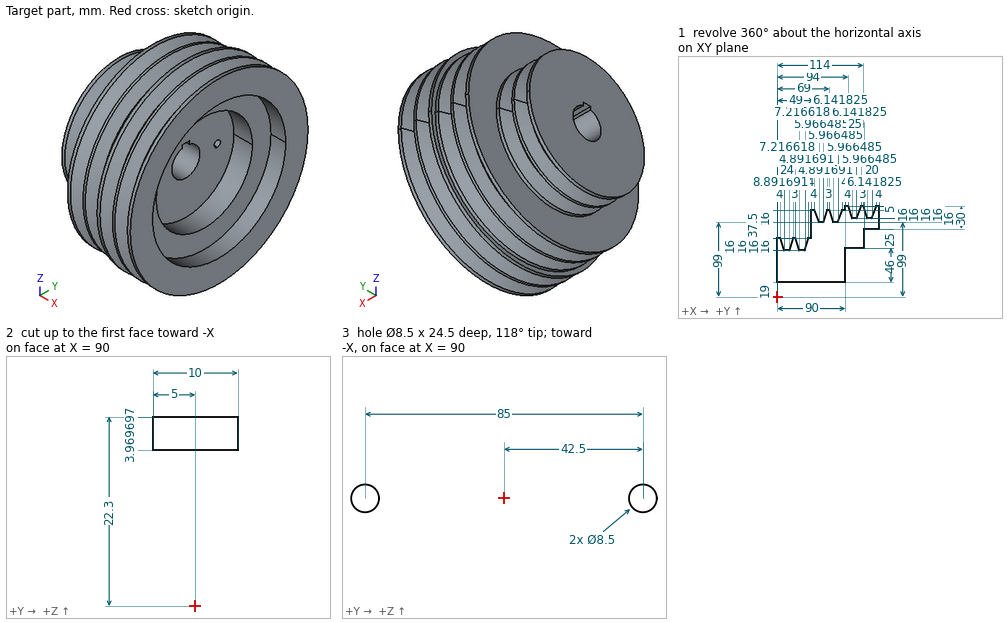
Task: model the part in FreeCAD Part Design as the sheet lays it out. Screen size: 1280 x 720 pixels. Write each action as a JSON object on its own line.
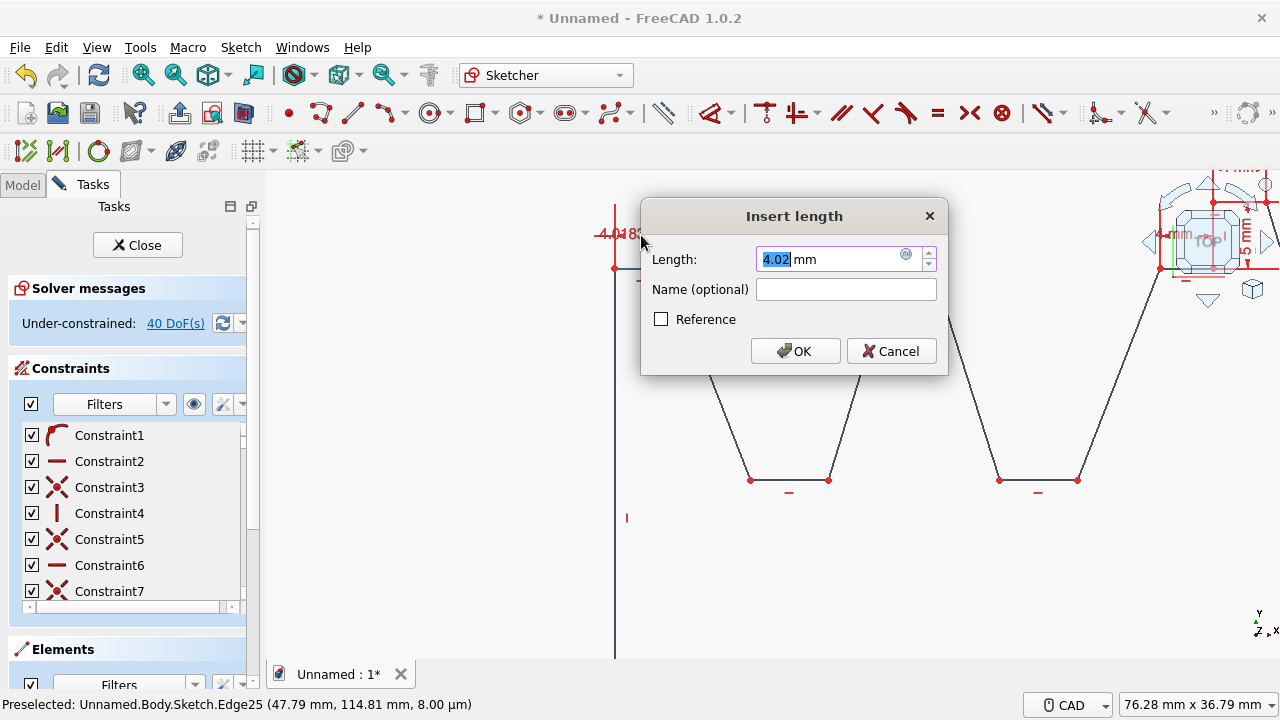
{"action": "type", "text": "4"}
{"action": "key", "text": "Return"}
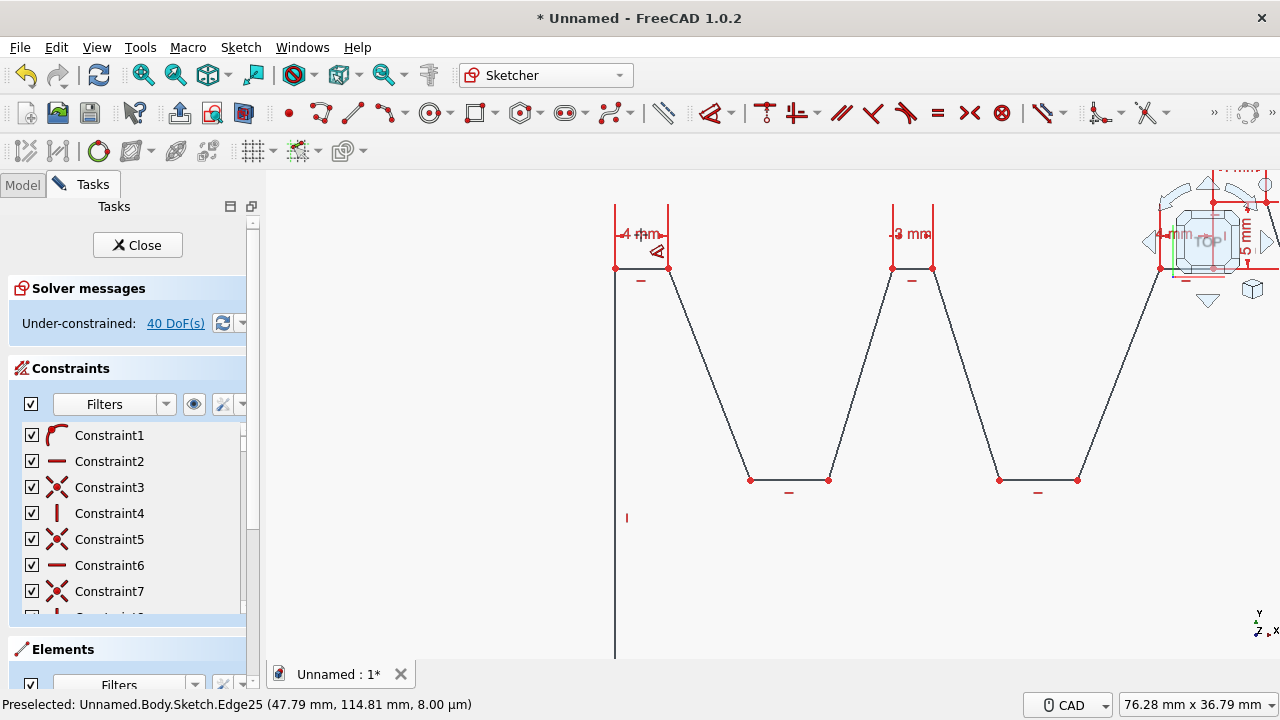
{"action": "scroll", "coordinate": [652, 267], "scroll_direction": "down", "scroll_amount": 8}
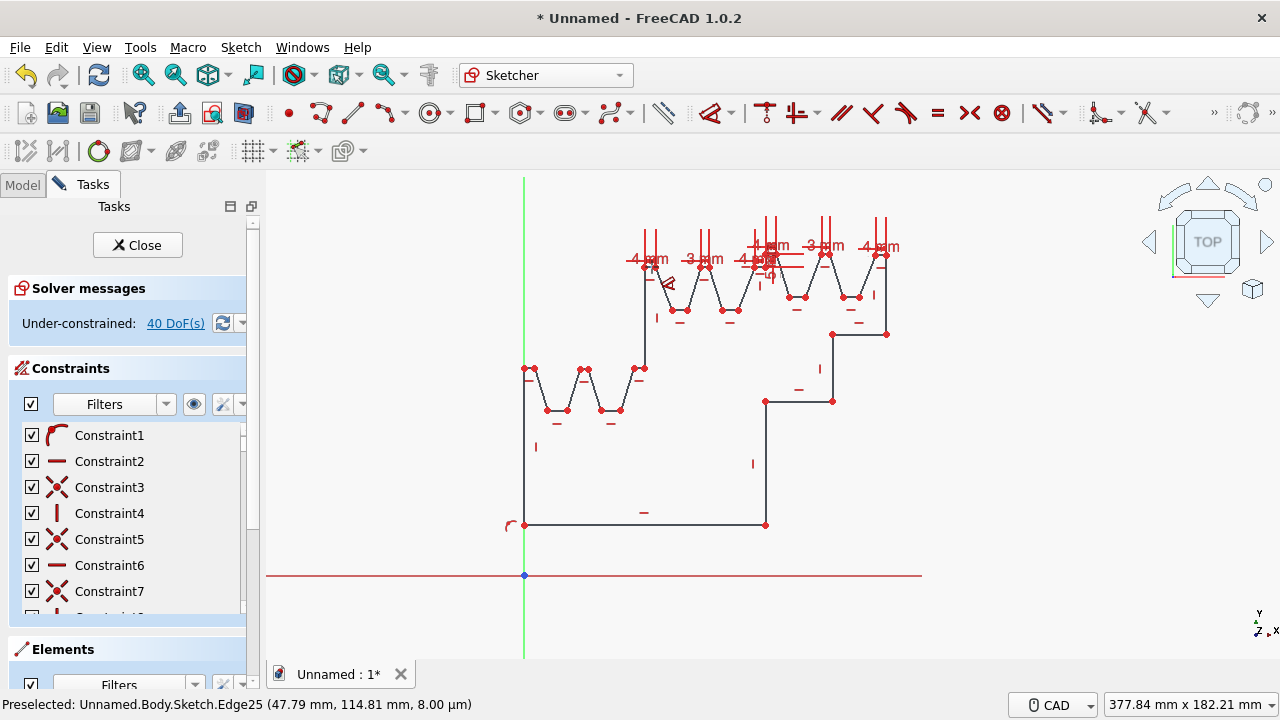
{"action": "scroll", "coordinate": [642, 368], "scroll_direction": "up", "scroll_amount": 8}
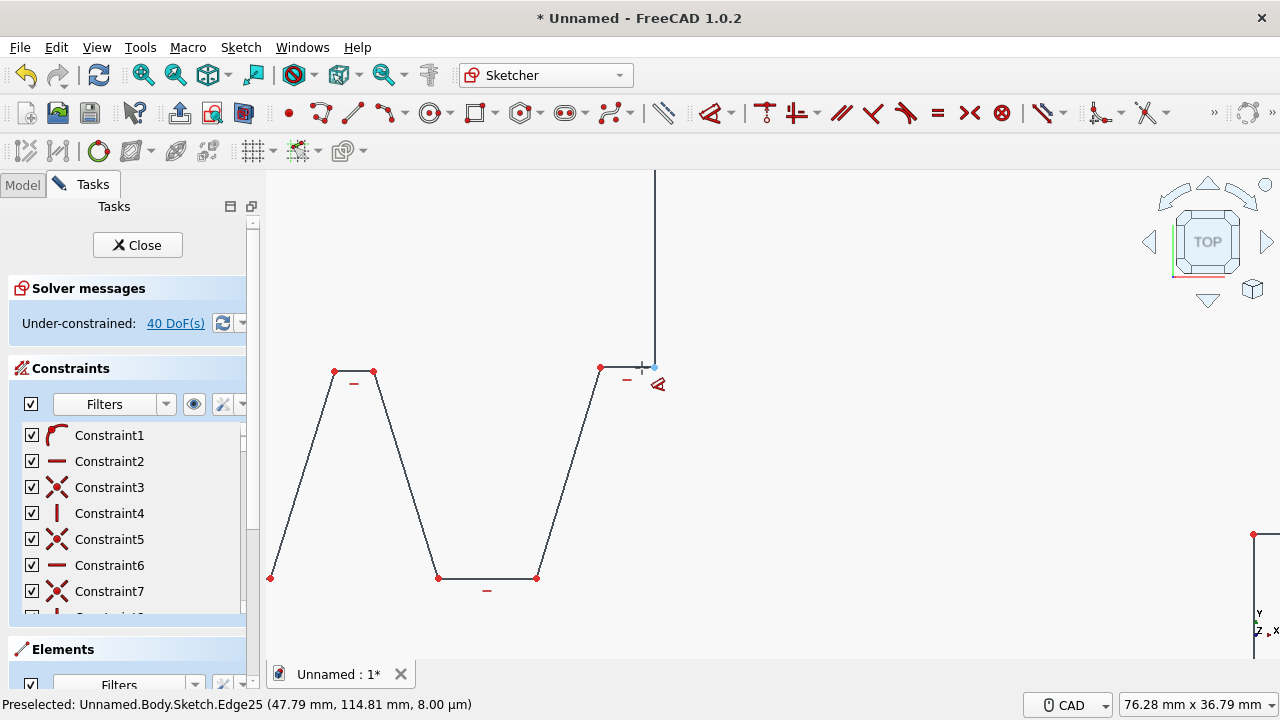
{"action": "left_click", "coordinate": [638, 367]}
{"action": "left_click", "coordinate": [628, 333]}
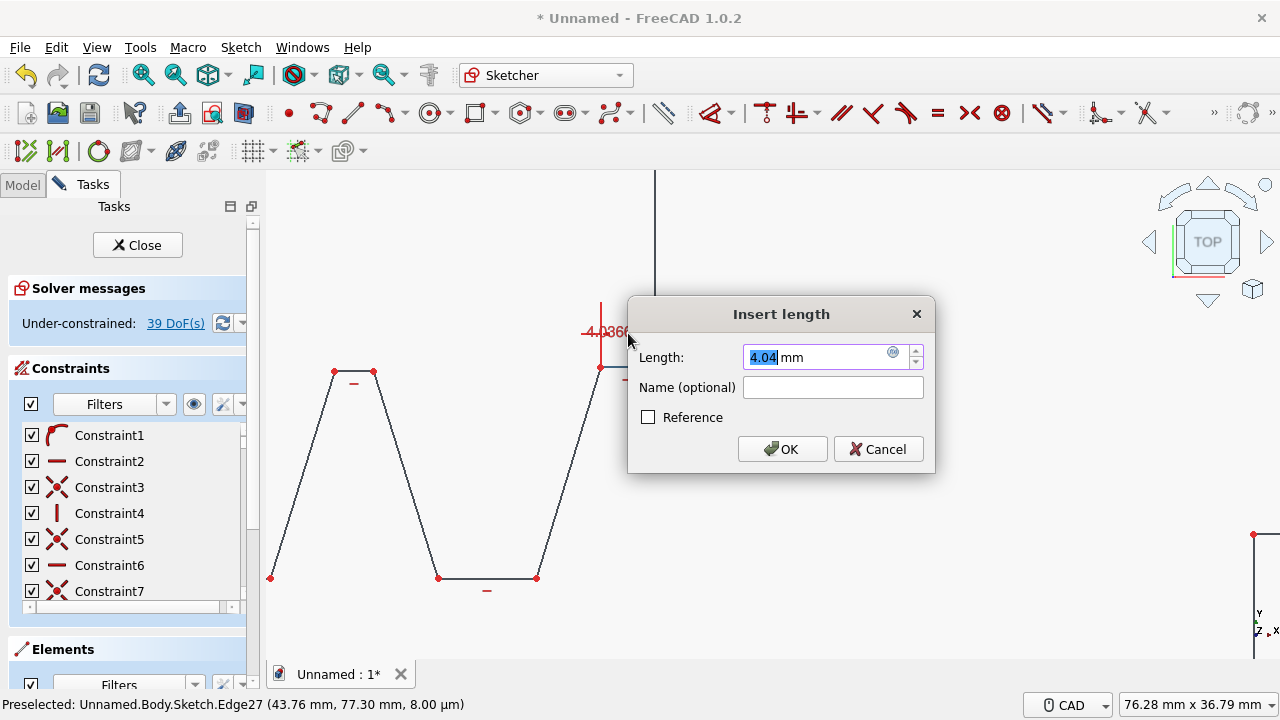
{"action": "type", "text": "4"}
{"action": "key", "text": "Return"}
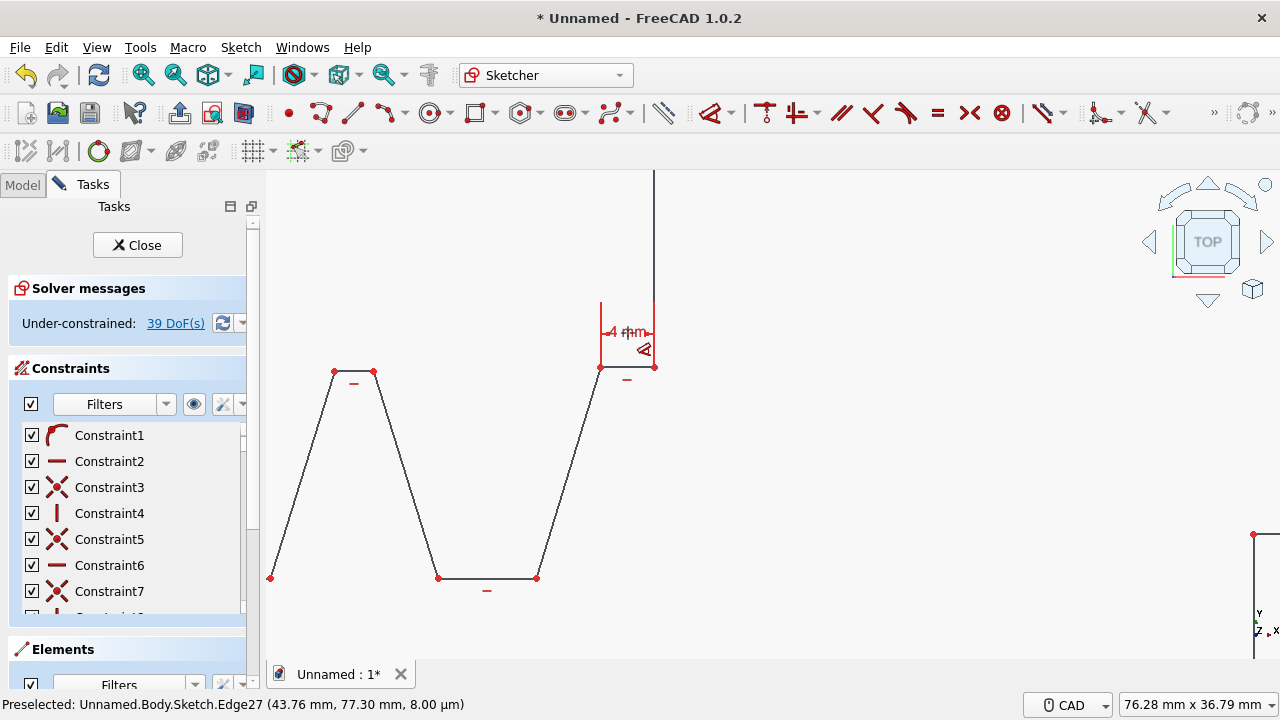
{"action": "left_click", "coordinate": [362, 371]}
{"action": "left_click", "coordinate": [354, 337]}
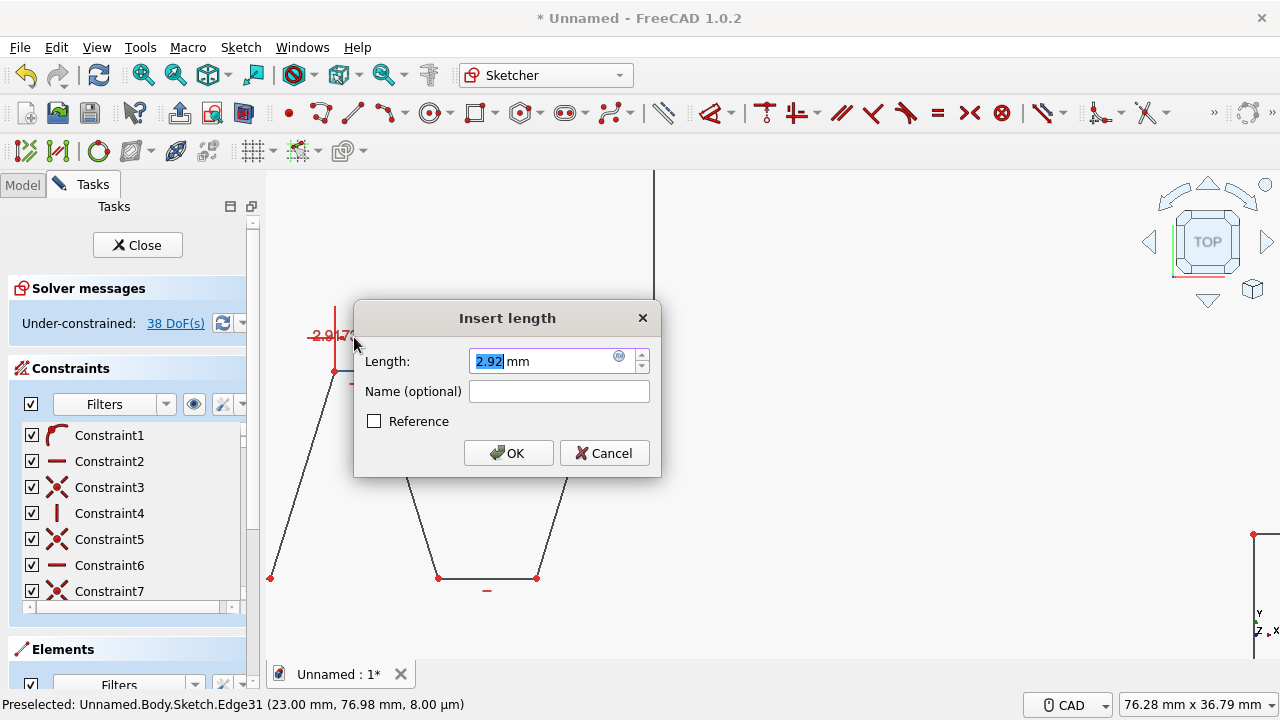
{"action": "type", "text": "3"}
{"action": "key", "text": "Return"}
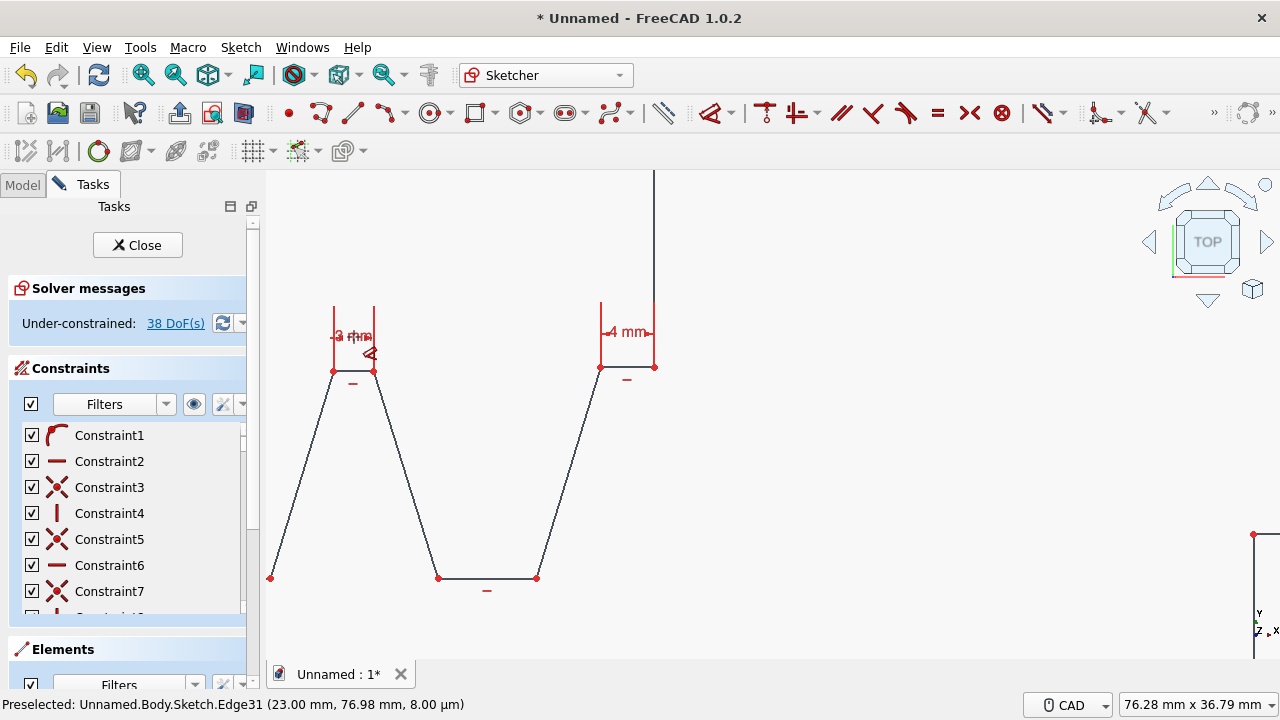
{"action": "scroll", "coordinate": [641, 368], "scroll_direction": "down", "scroll_amount": 8}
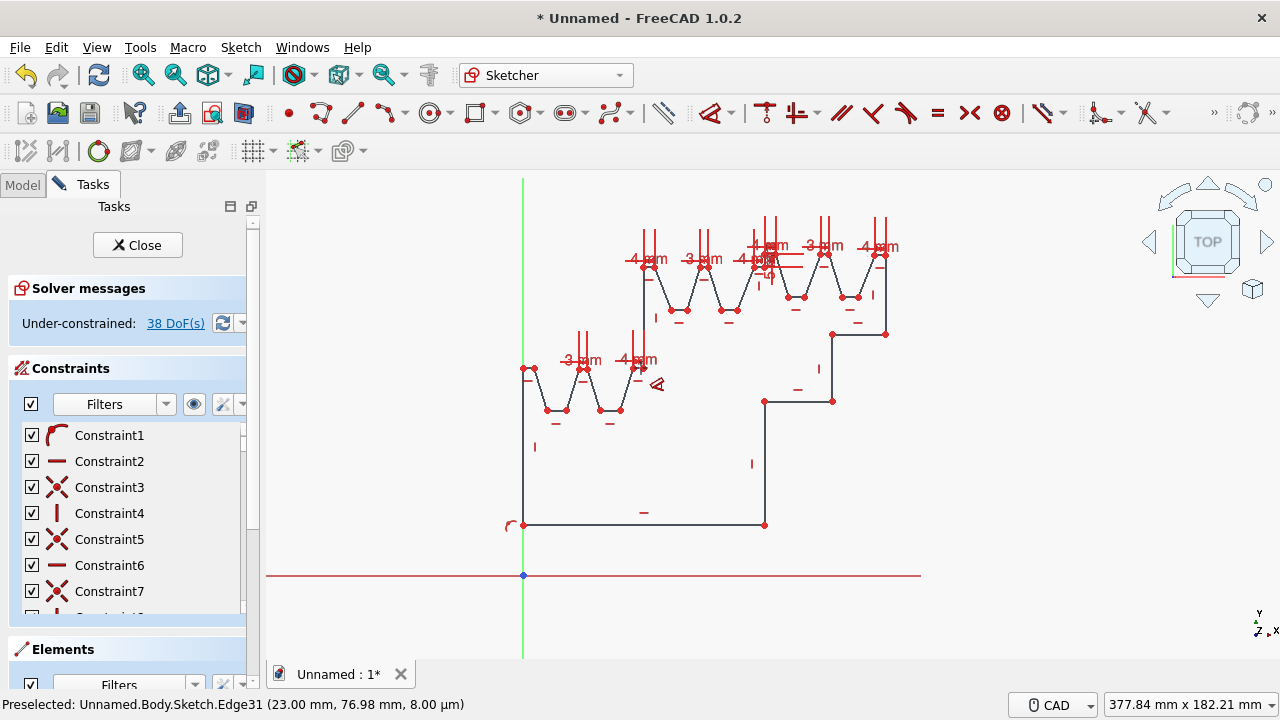
{"action": "scroll", "coordinate": [531, 368], "scroll_direction": "up", "scroll_amount": 8}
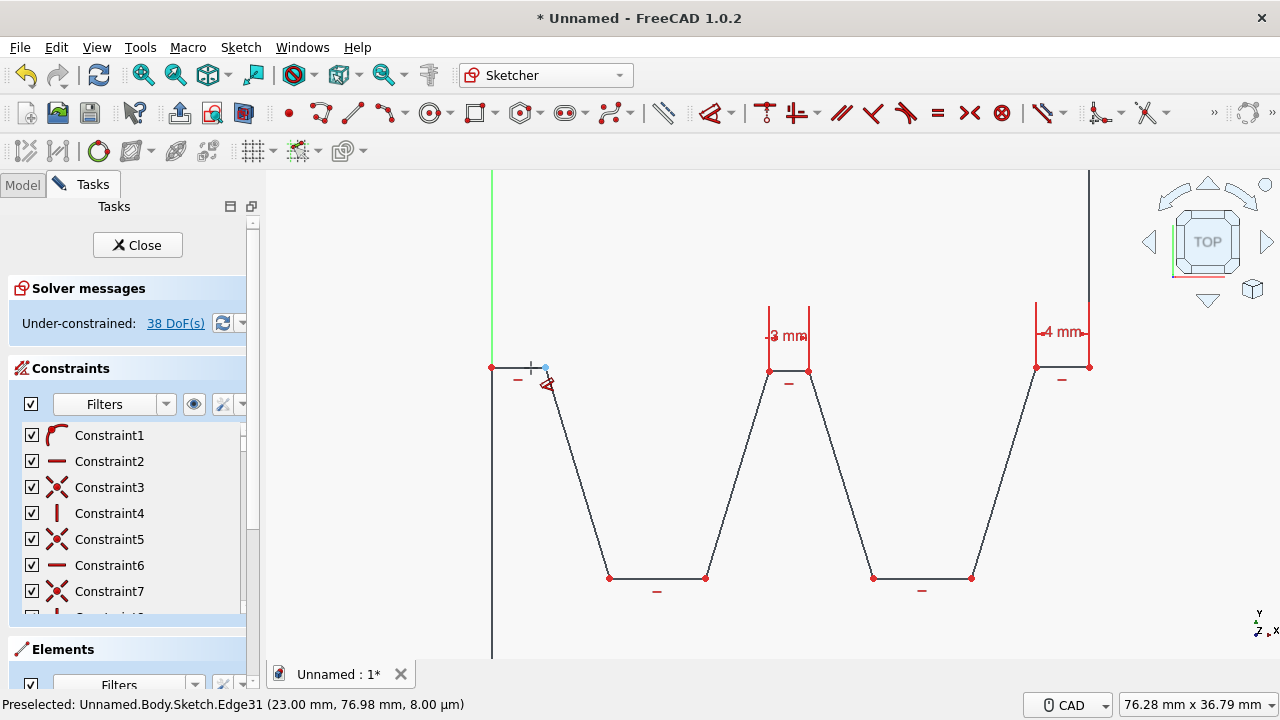
{"action": "left_click", "coordinate": [529, 368]}
{"action": "left_click", "coordinate": [518, 334]}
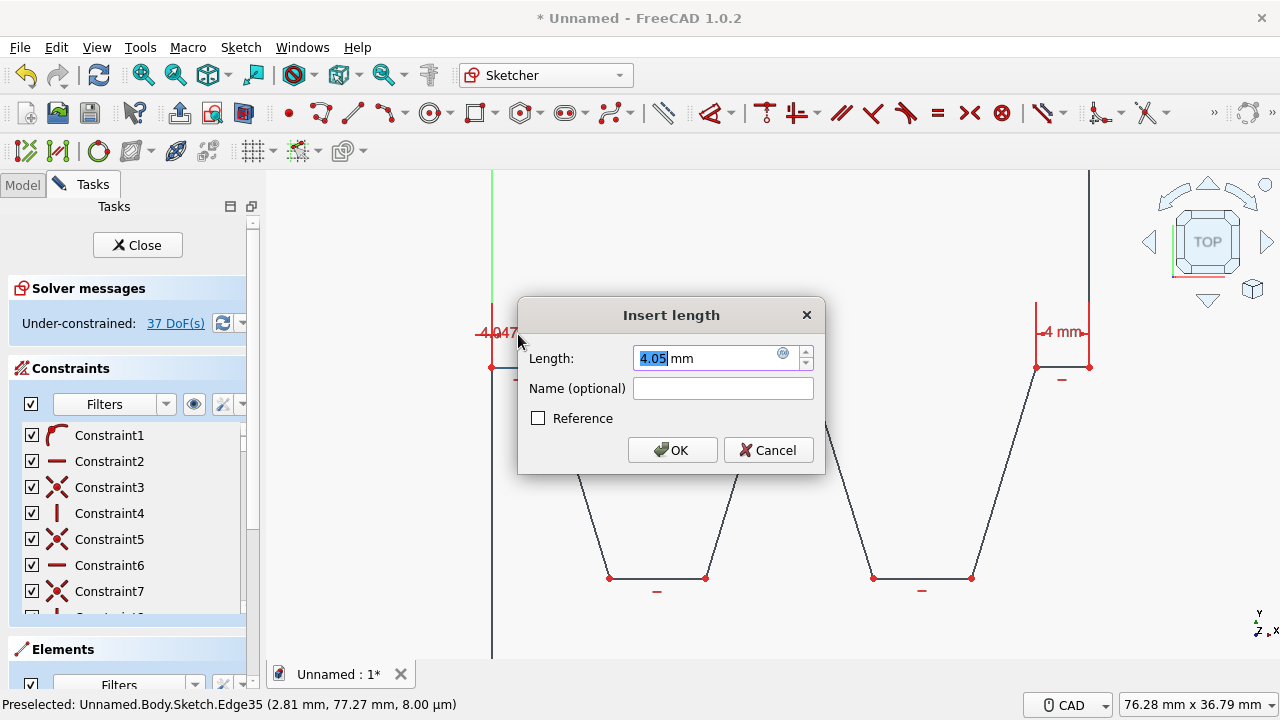
{"action": "type", "text": "4"}
{"action": "key", "text": "Return"}